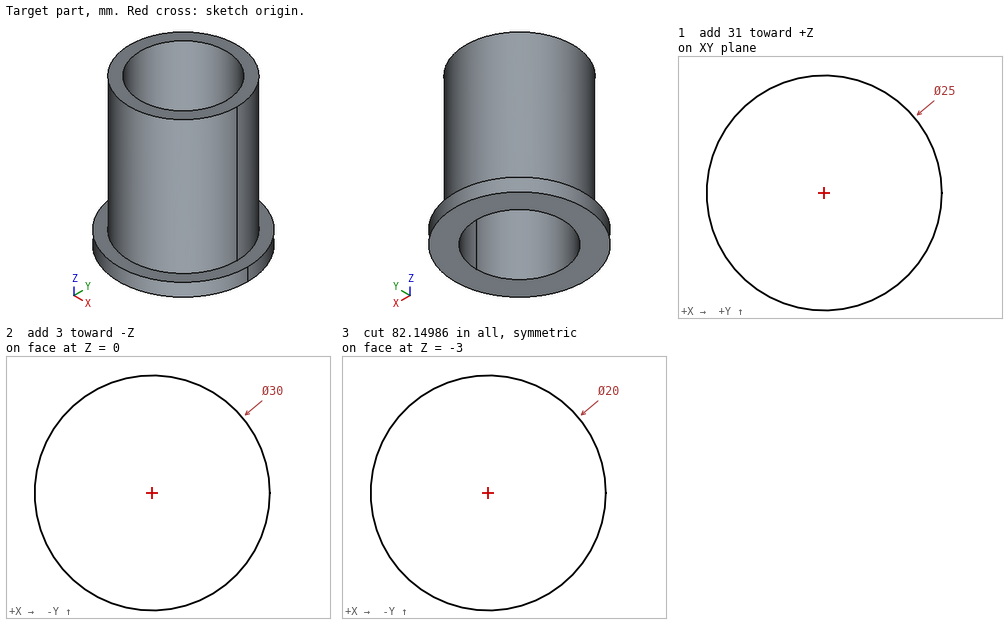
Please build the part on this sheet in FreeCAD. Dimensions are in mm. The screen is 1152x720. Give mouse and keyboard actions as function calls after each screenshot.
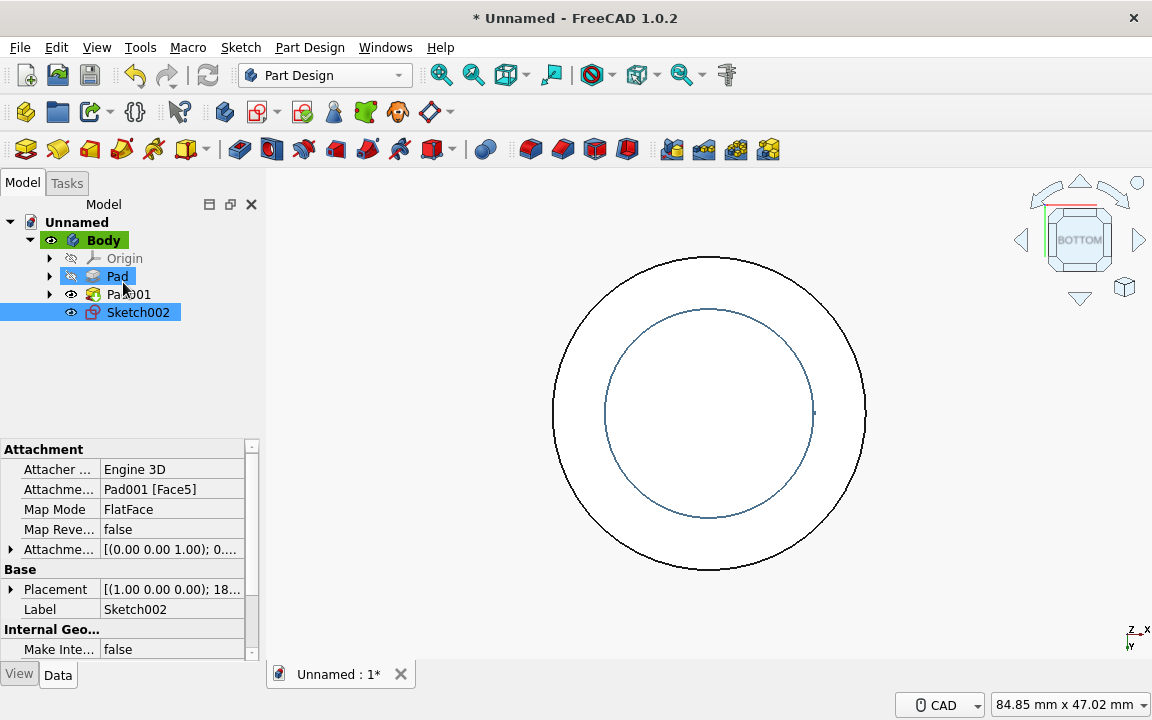
click(240, 150)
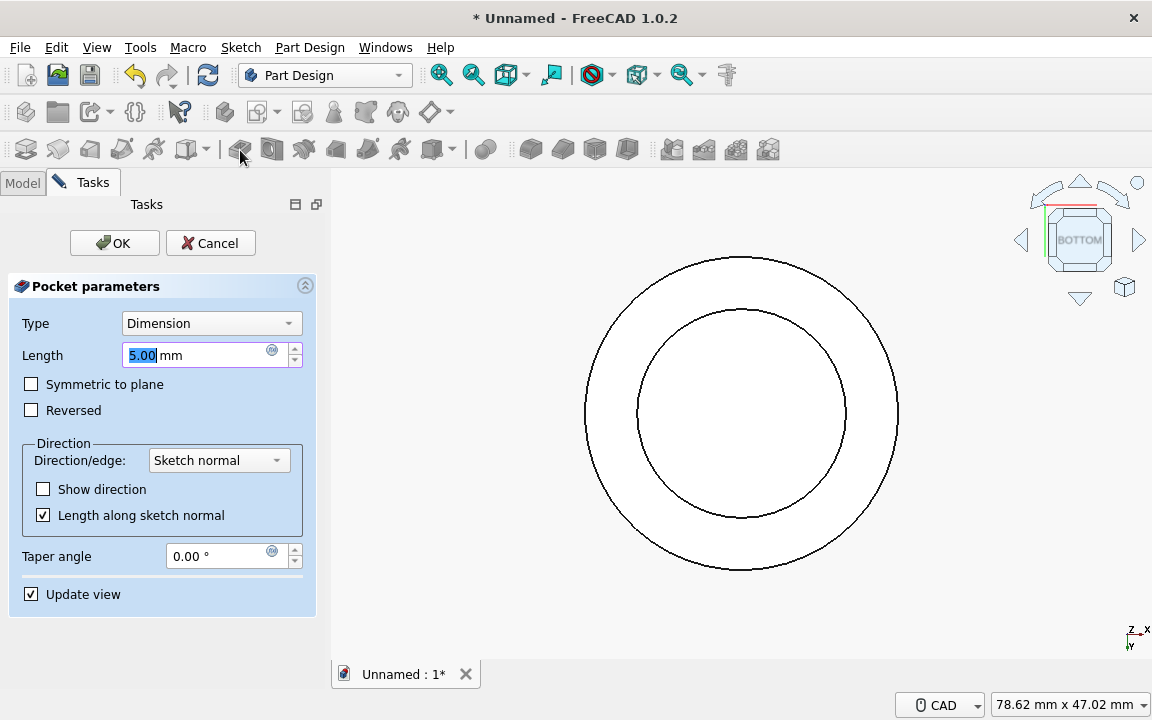
text(82.14986)
key(Tab)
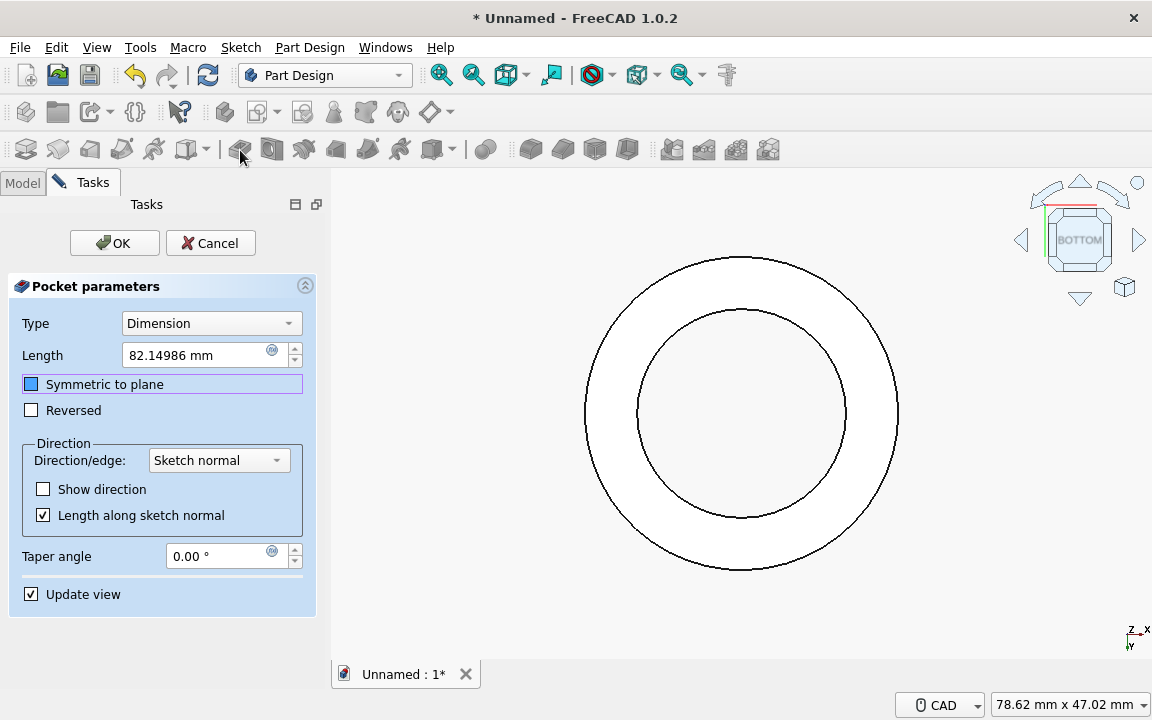
click(30, 384)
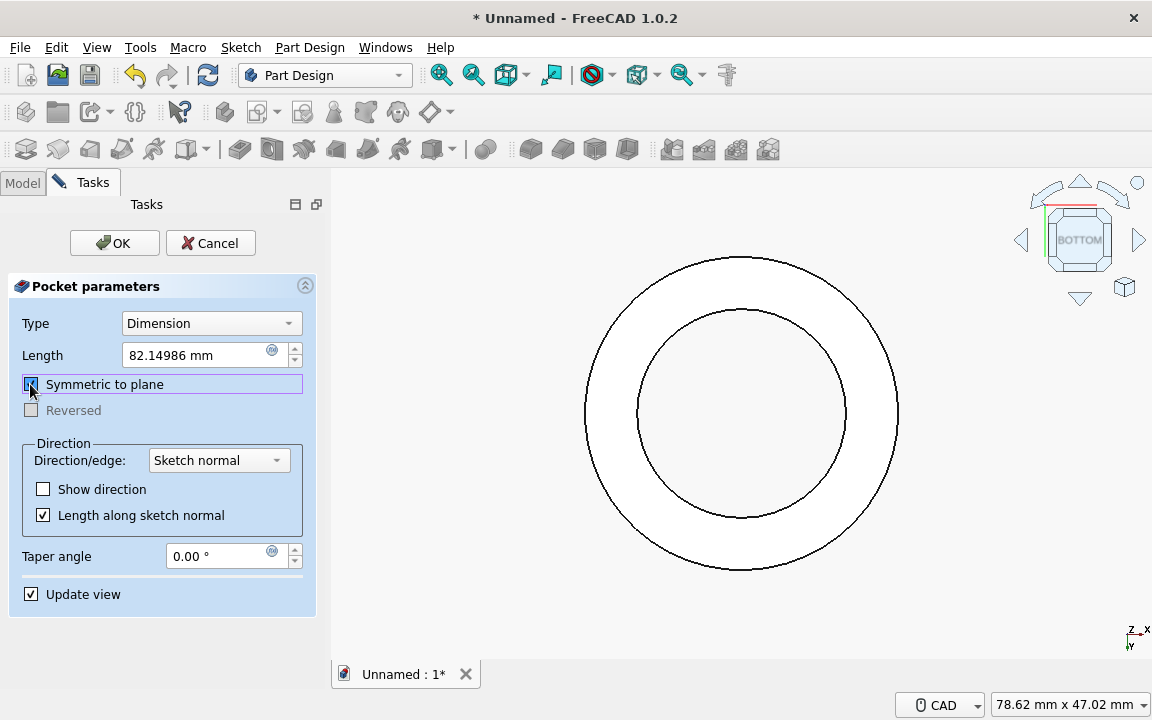
click(115, 243)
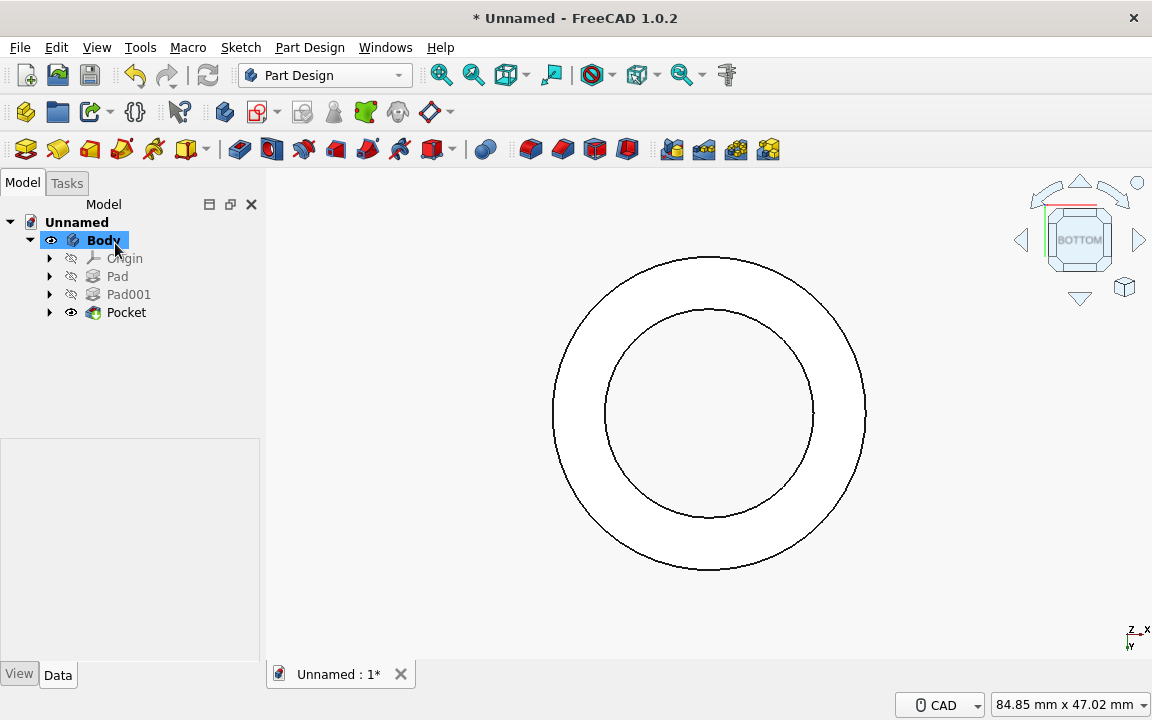
key(0)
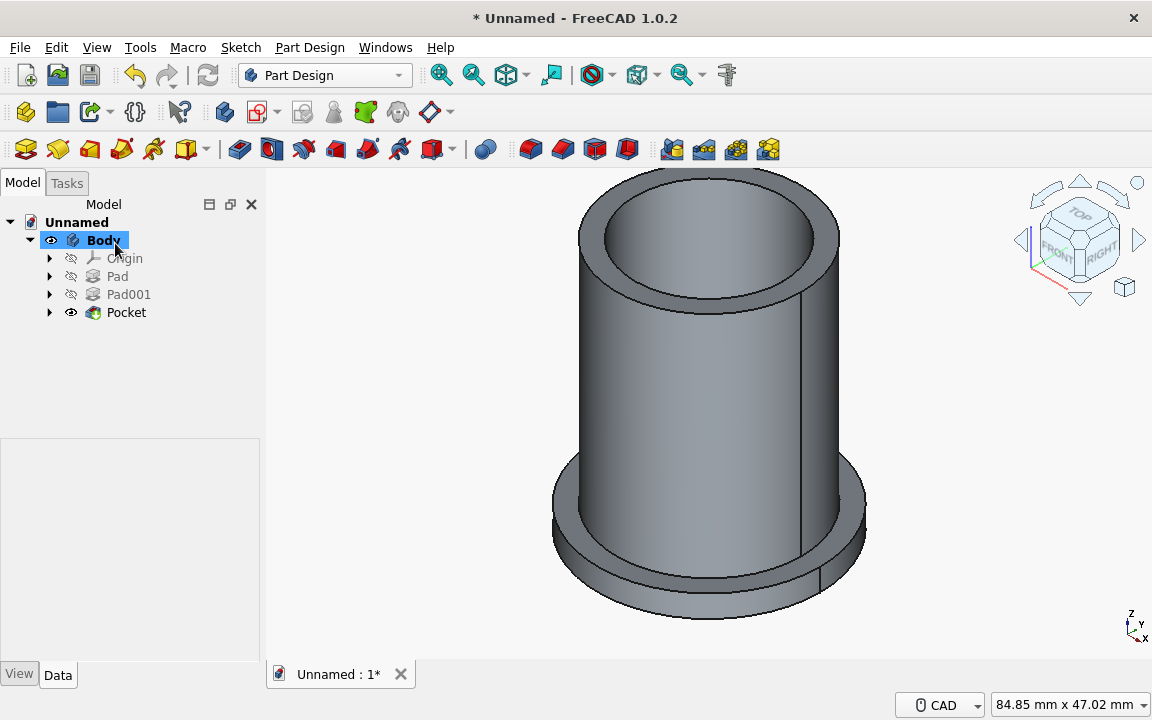
click(442, 76)